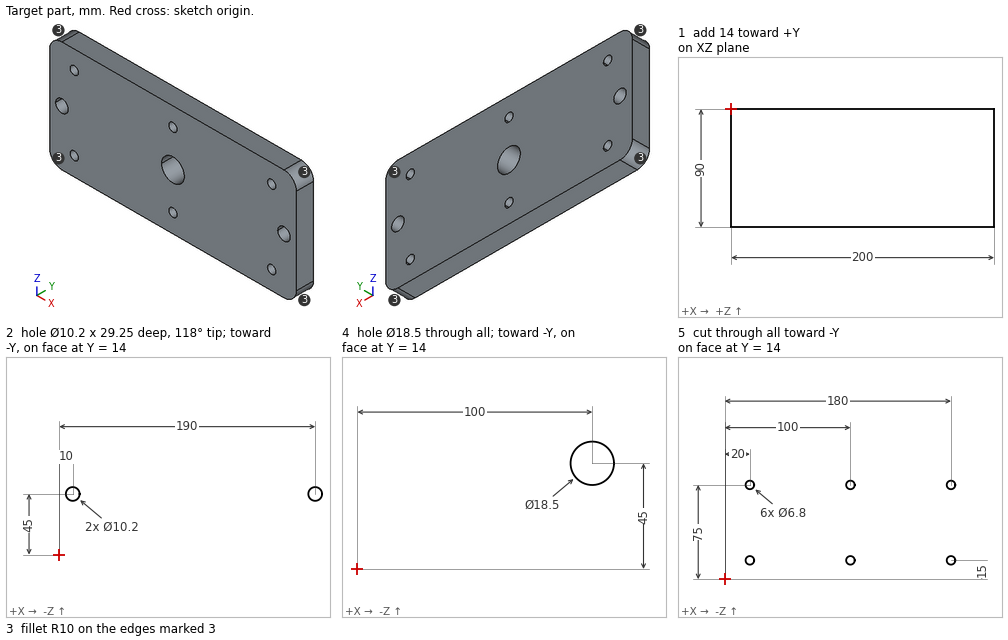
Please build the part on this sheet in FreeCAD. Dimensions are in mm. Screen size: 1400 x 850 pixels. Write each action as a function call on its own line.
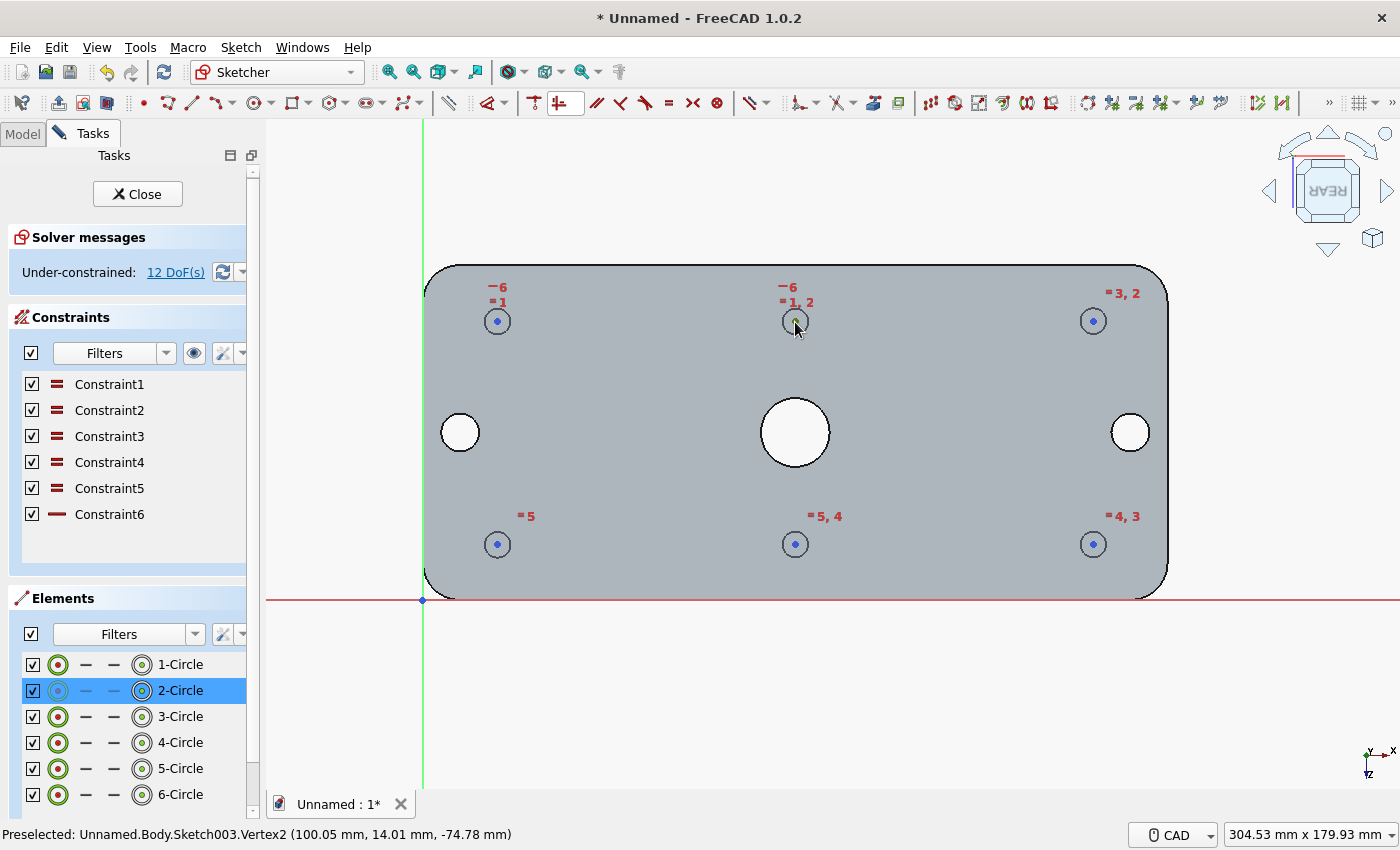
click(1093, 321)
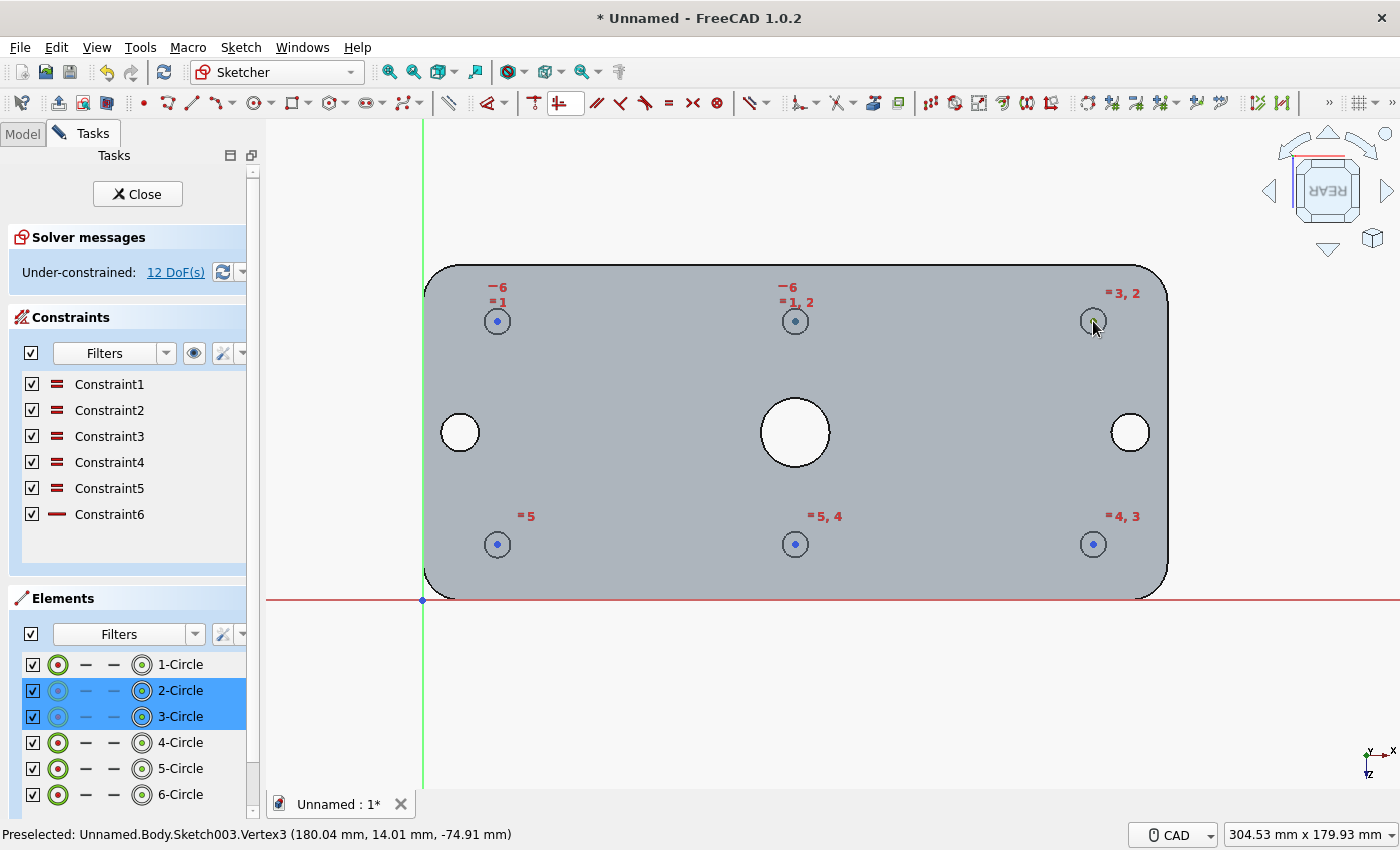
click(578, 104)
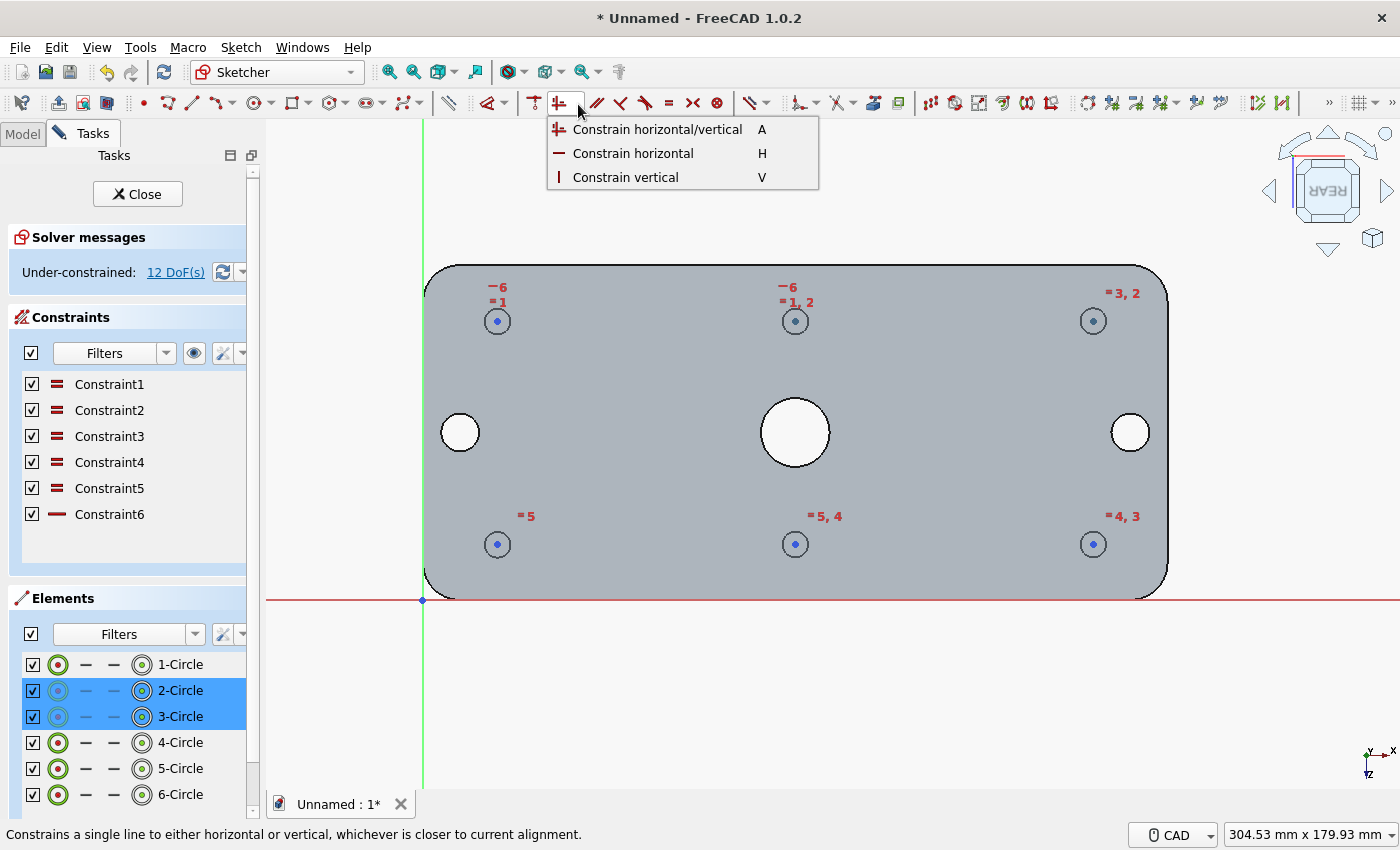
click(683, 153)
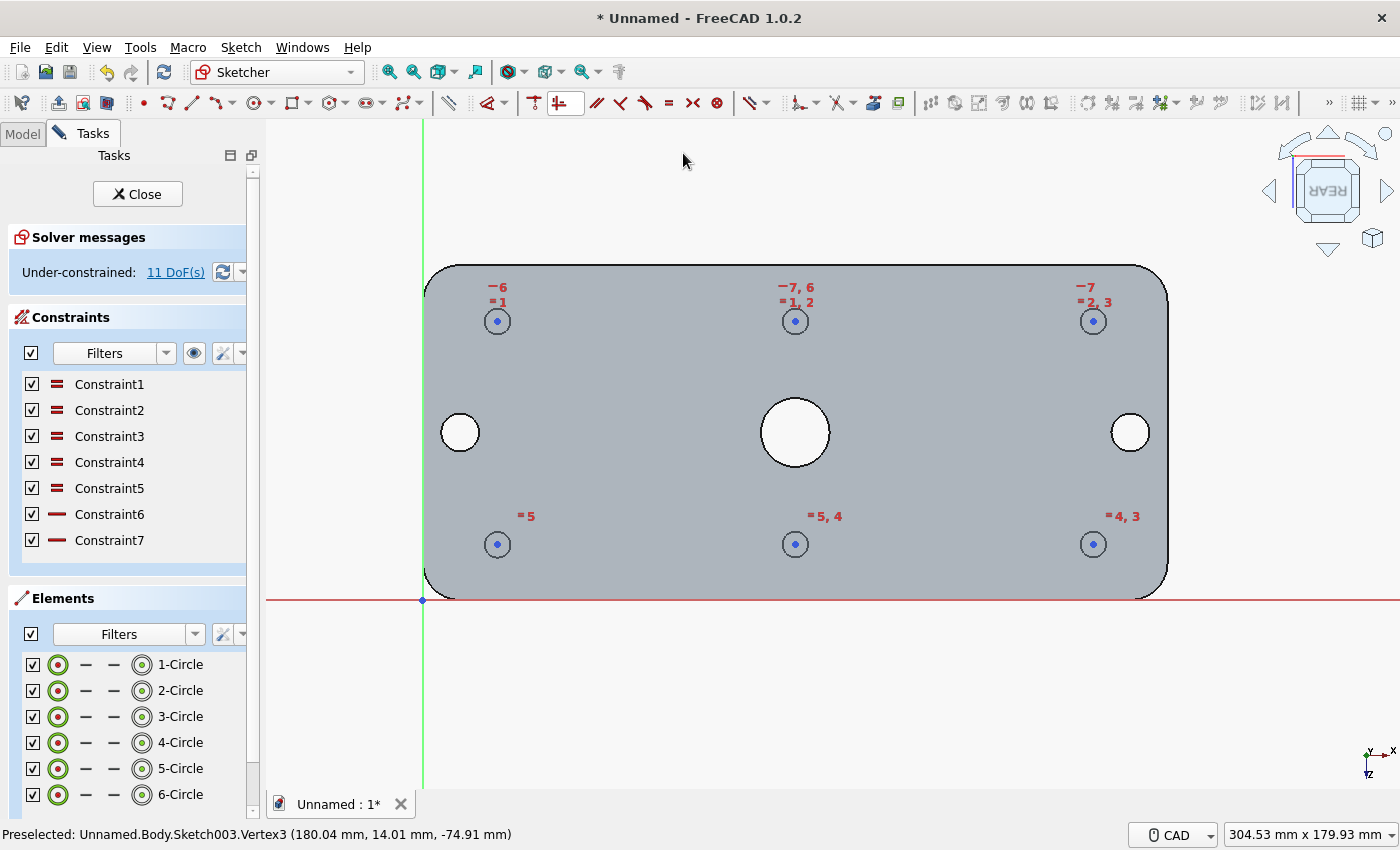
click(1093, 322)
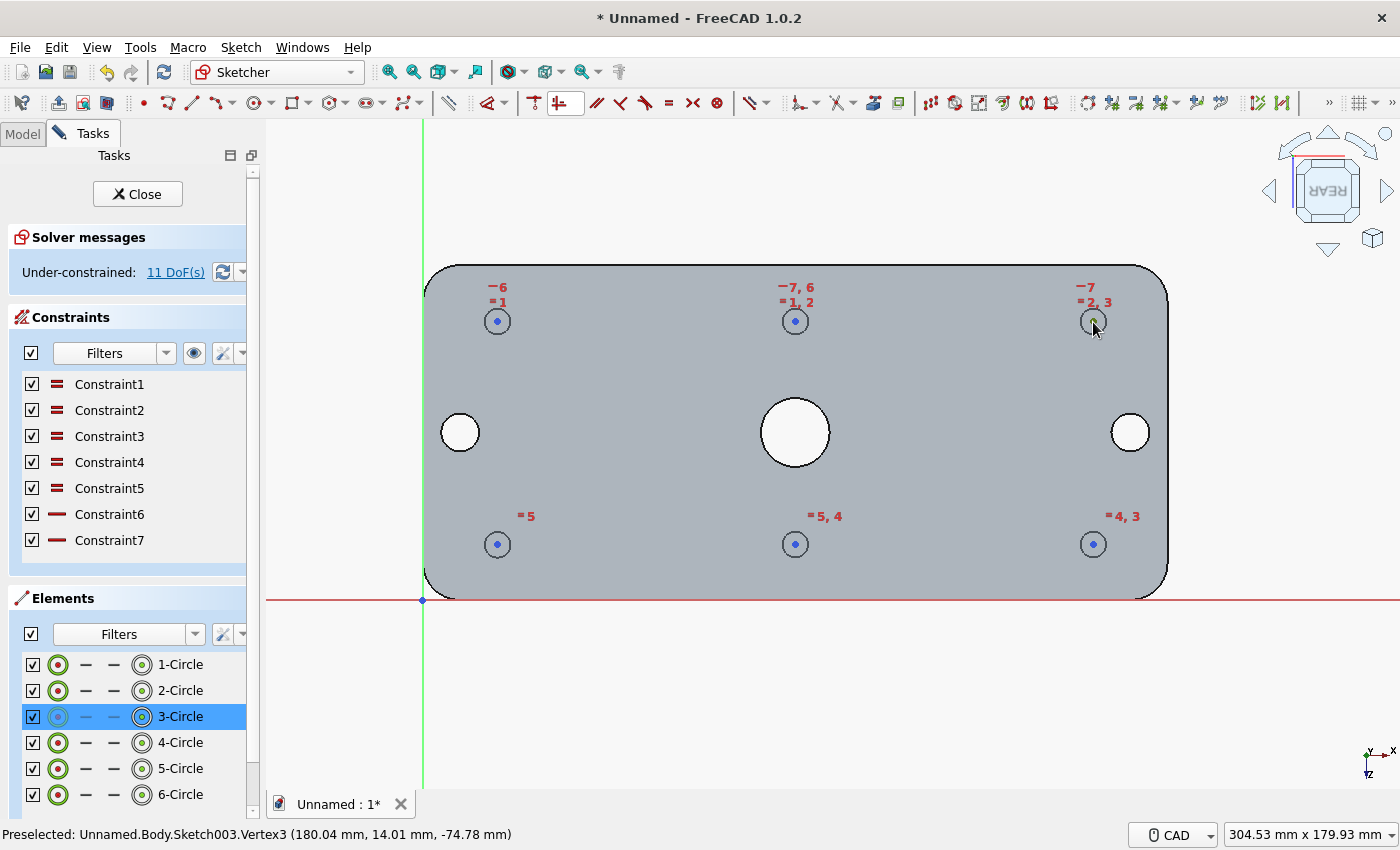
click(1093, 545)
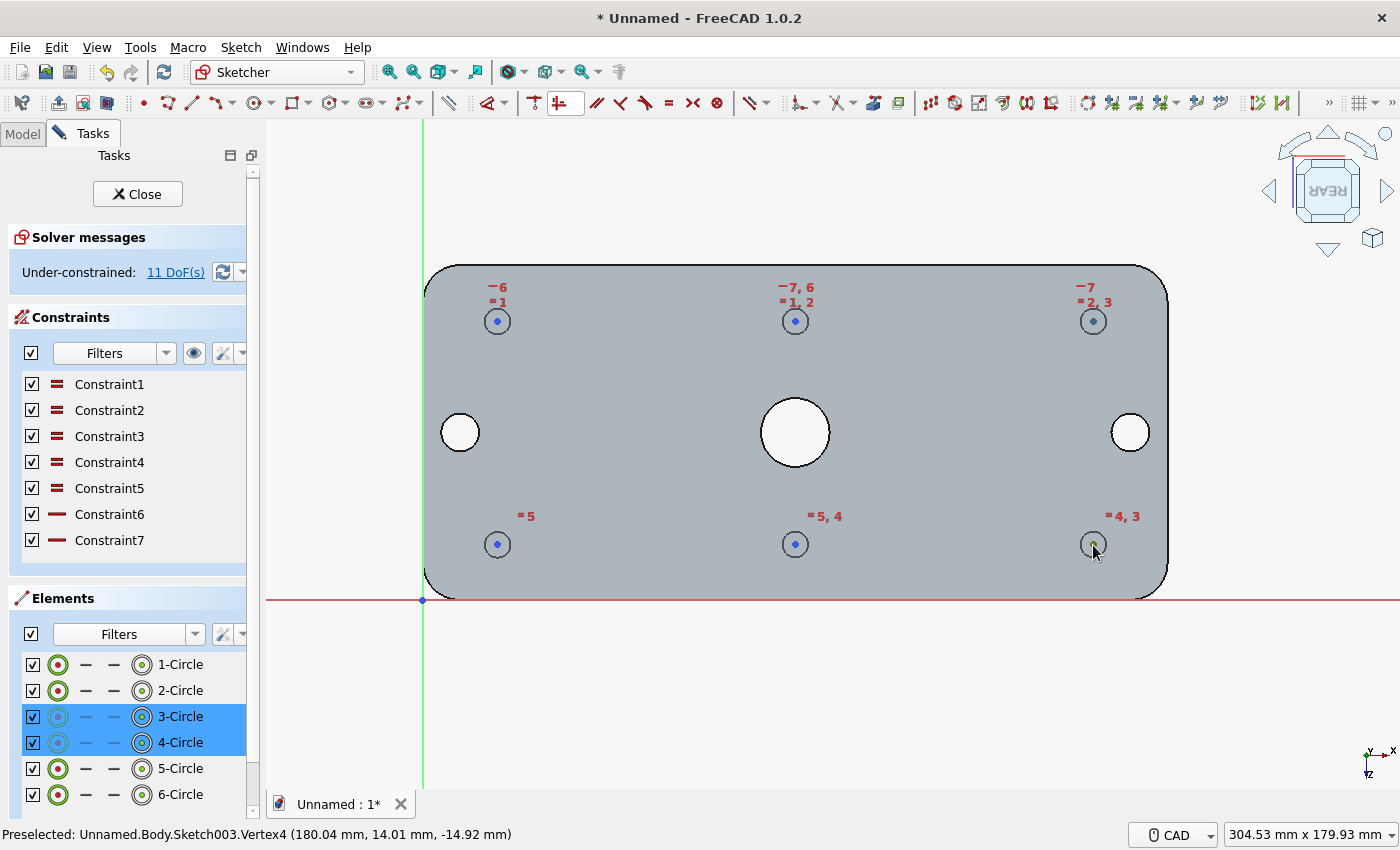
key(v)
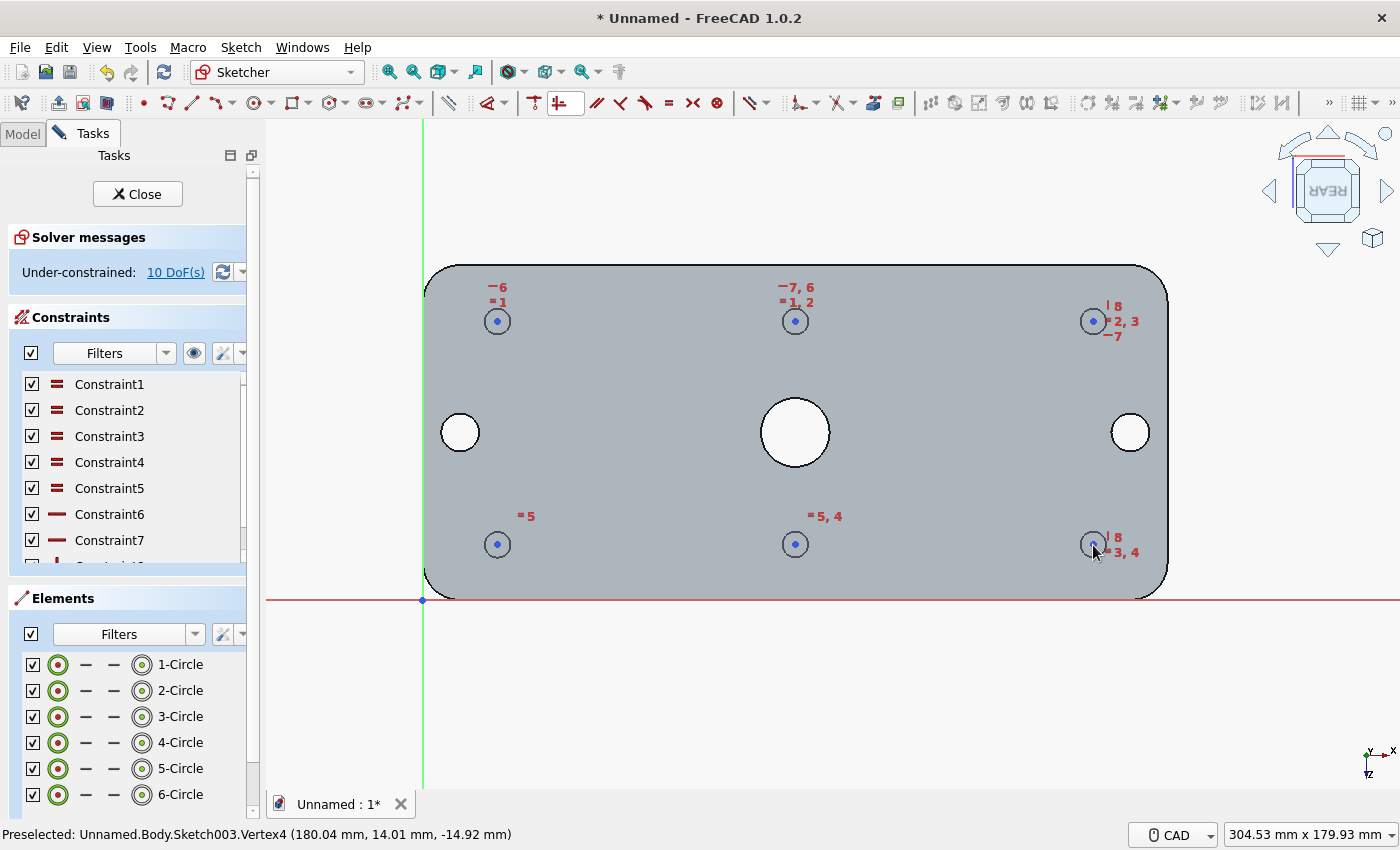
click(795, 322)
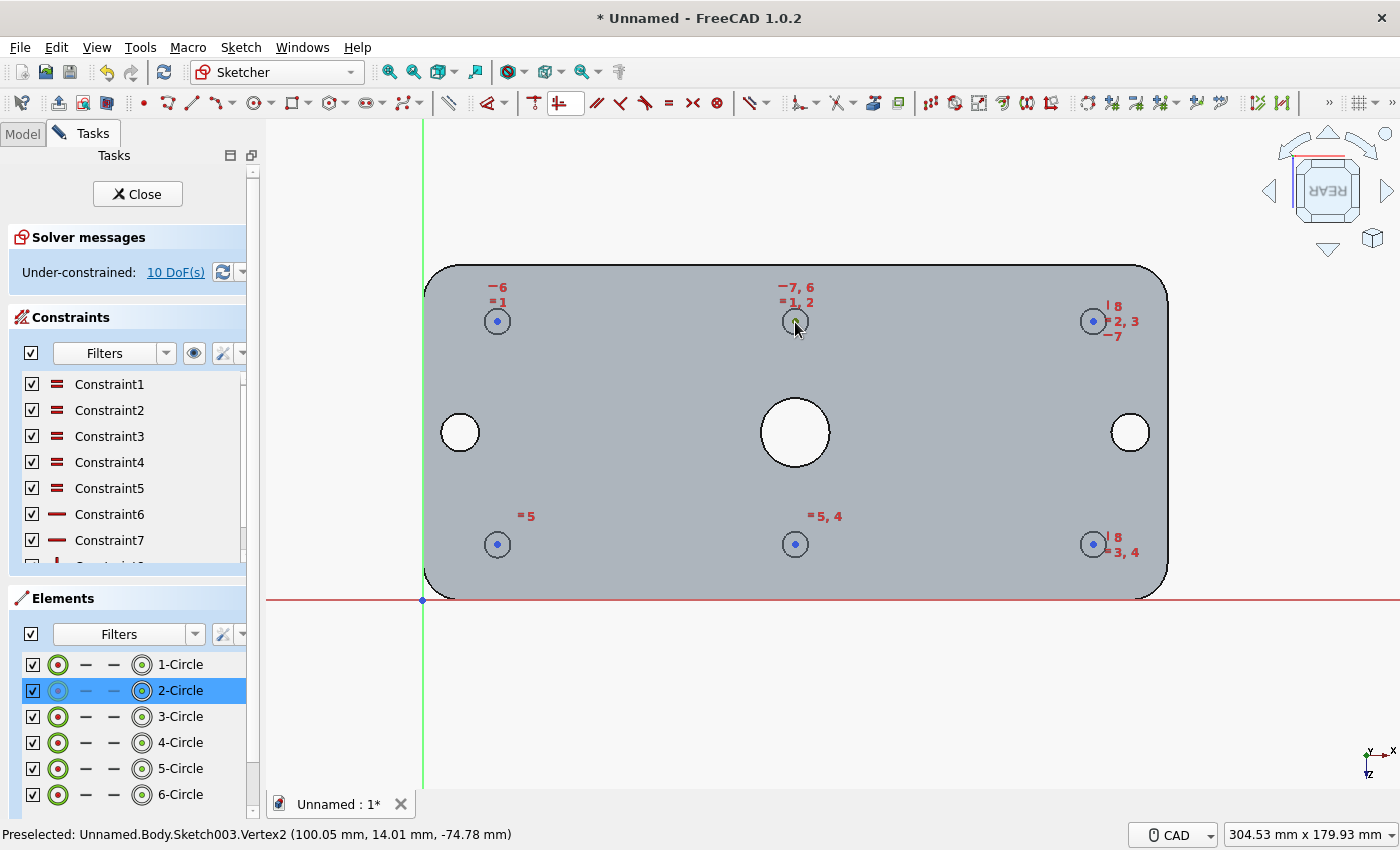
click(795, 545)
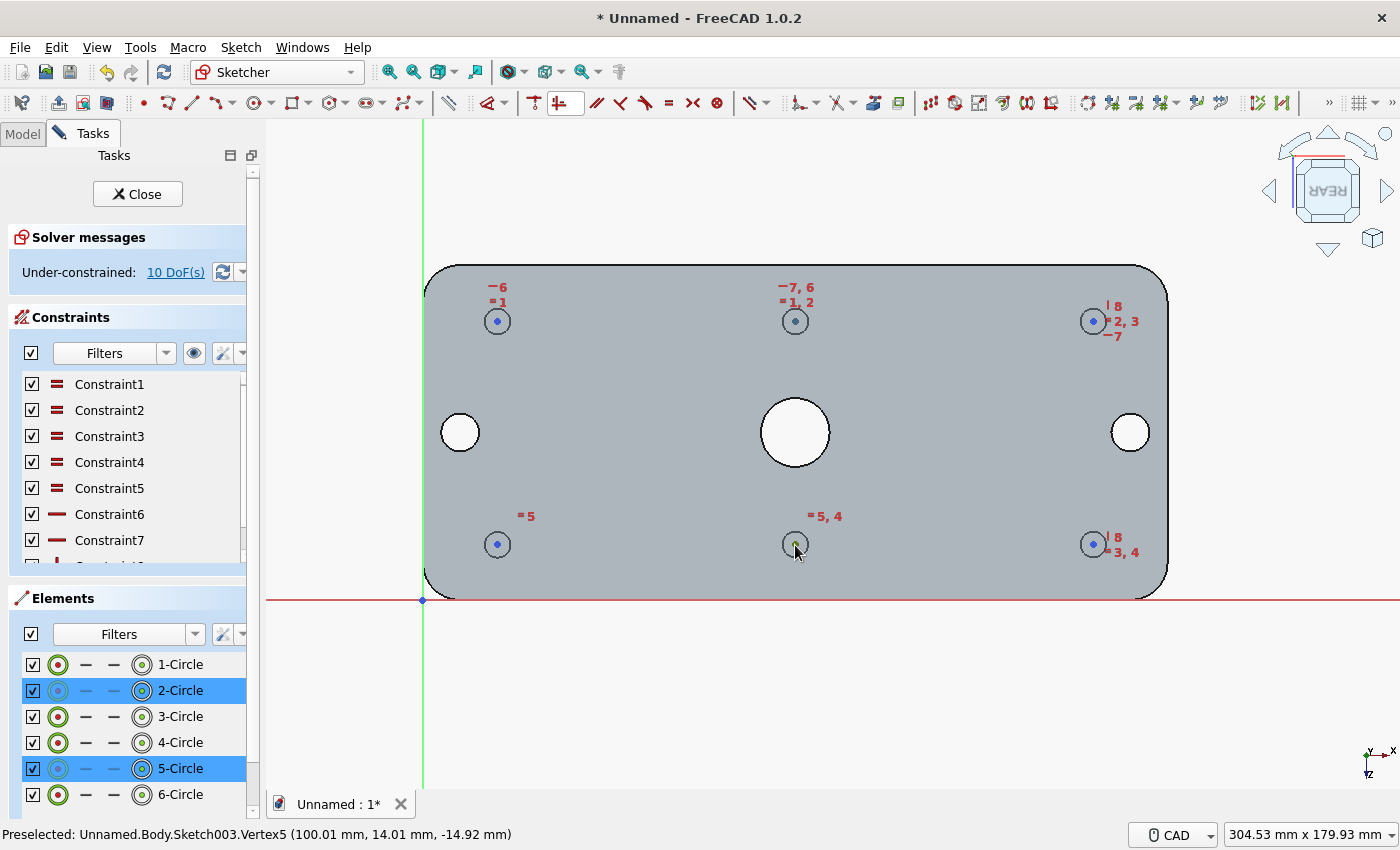
key(v)